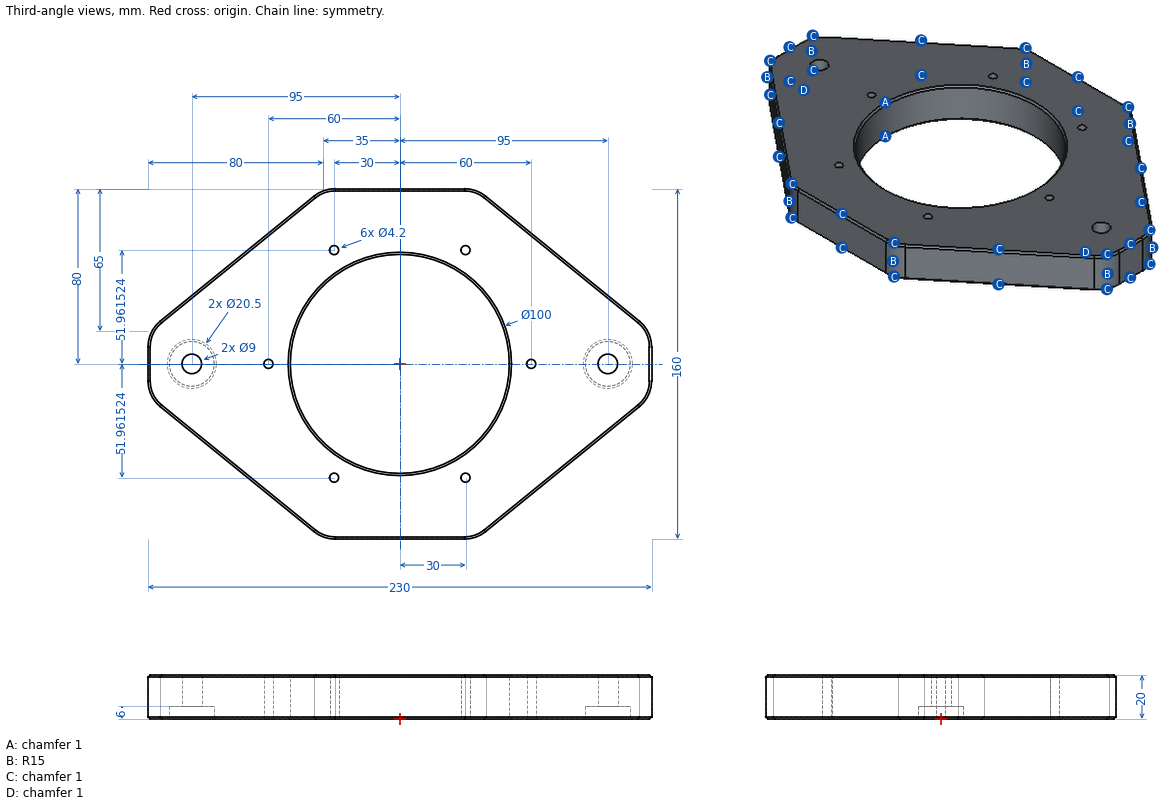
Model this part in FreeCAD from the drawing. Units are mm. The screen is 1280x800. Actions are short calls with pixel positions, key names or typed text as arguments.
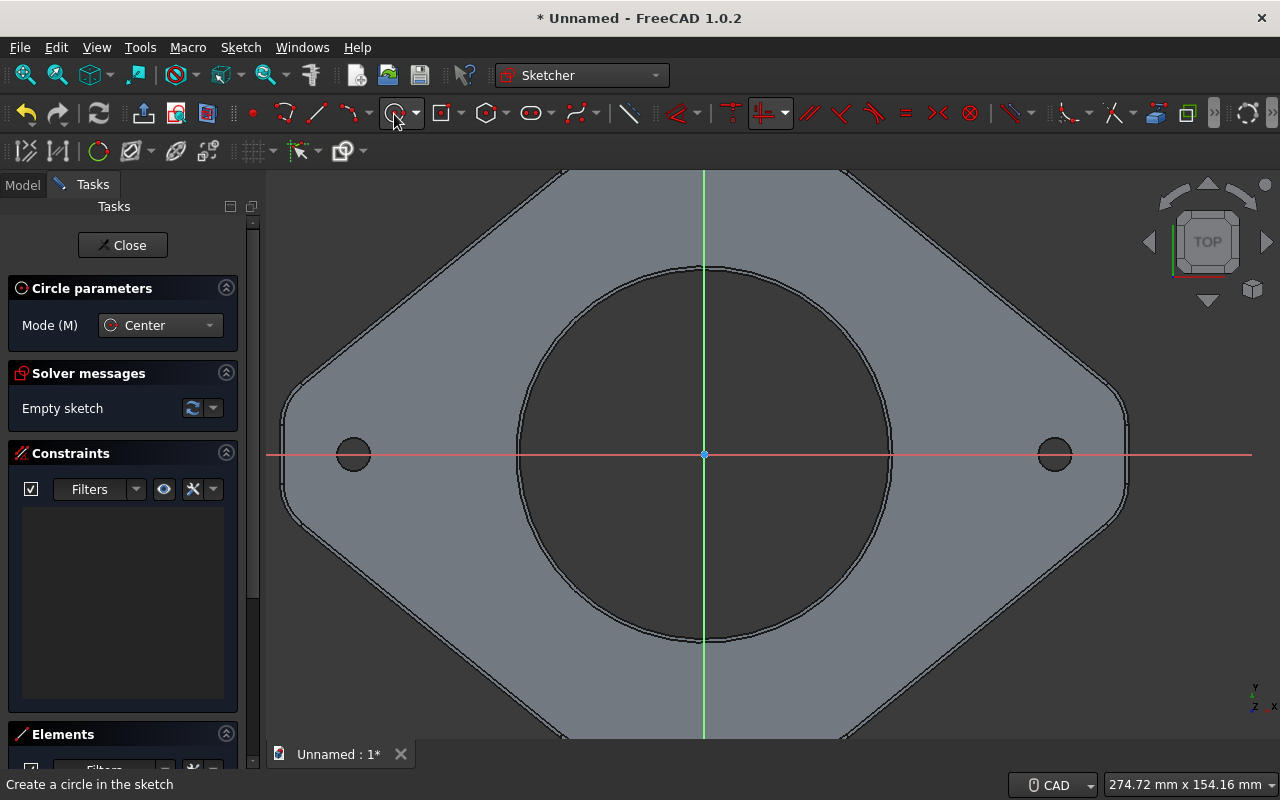
scroll(594, 263, up, 6)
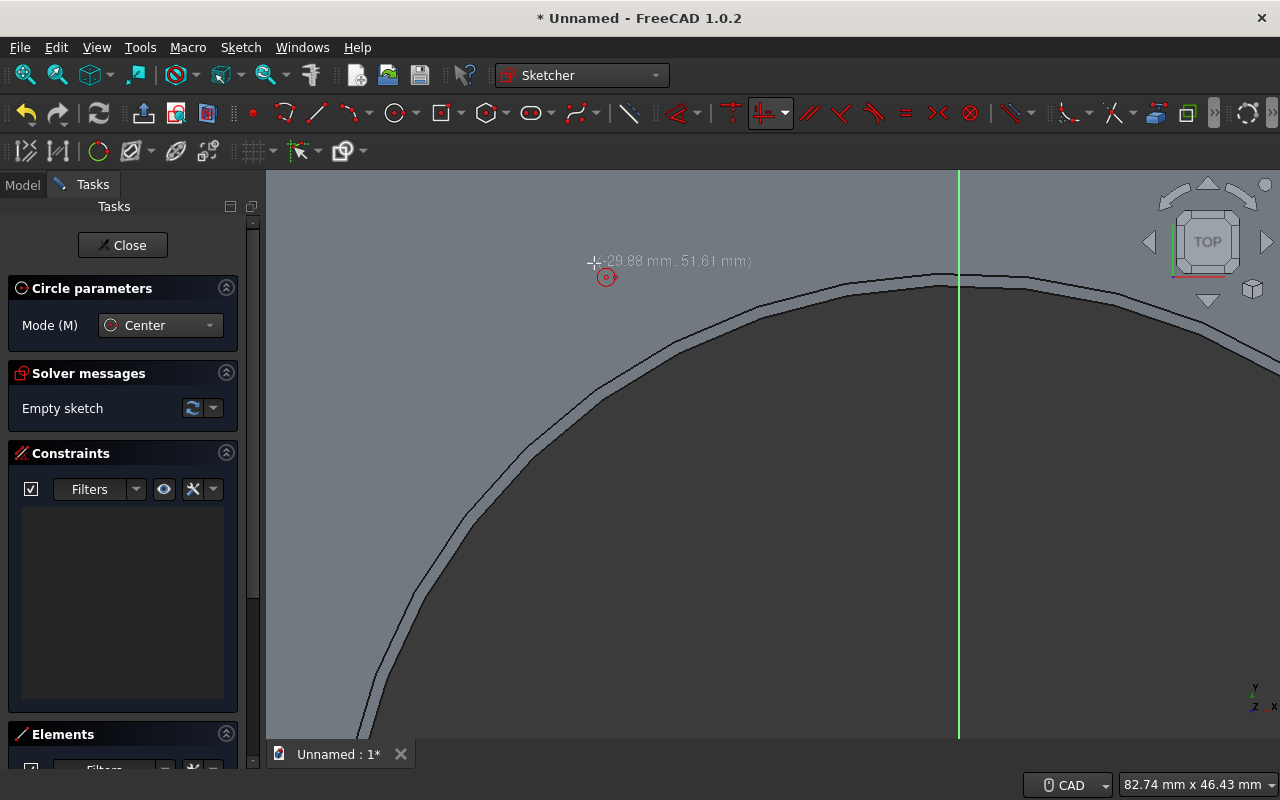
click(592, 262)
move(610, 243)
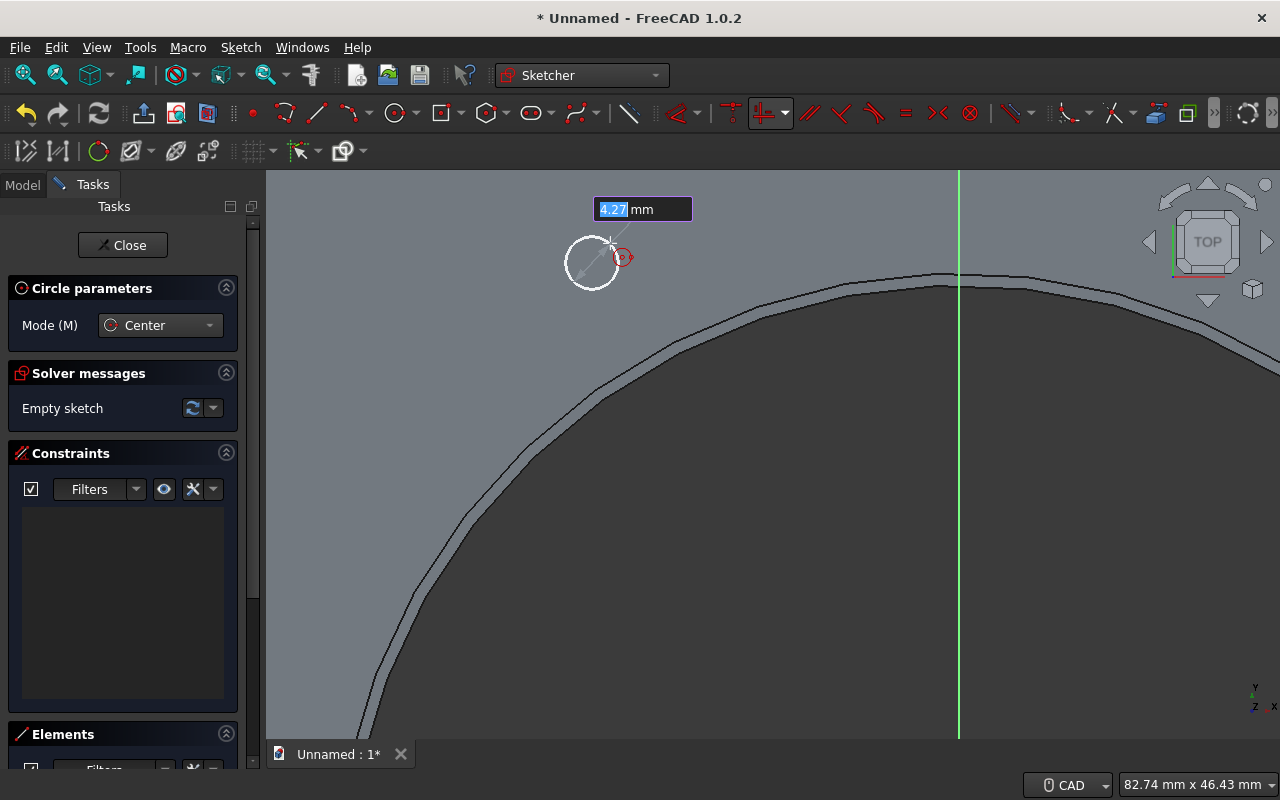
text(4.2)
key(Return)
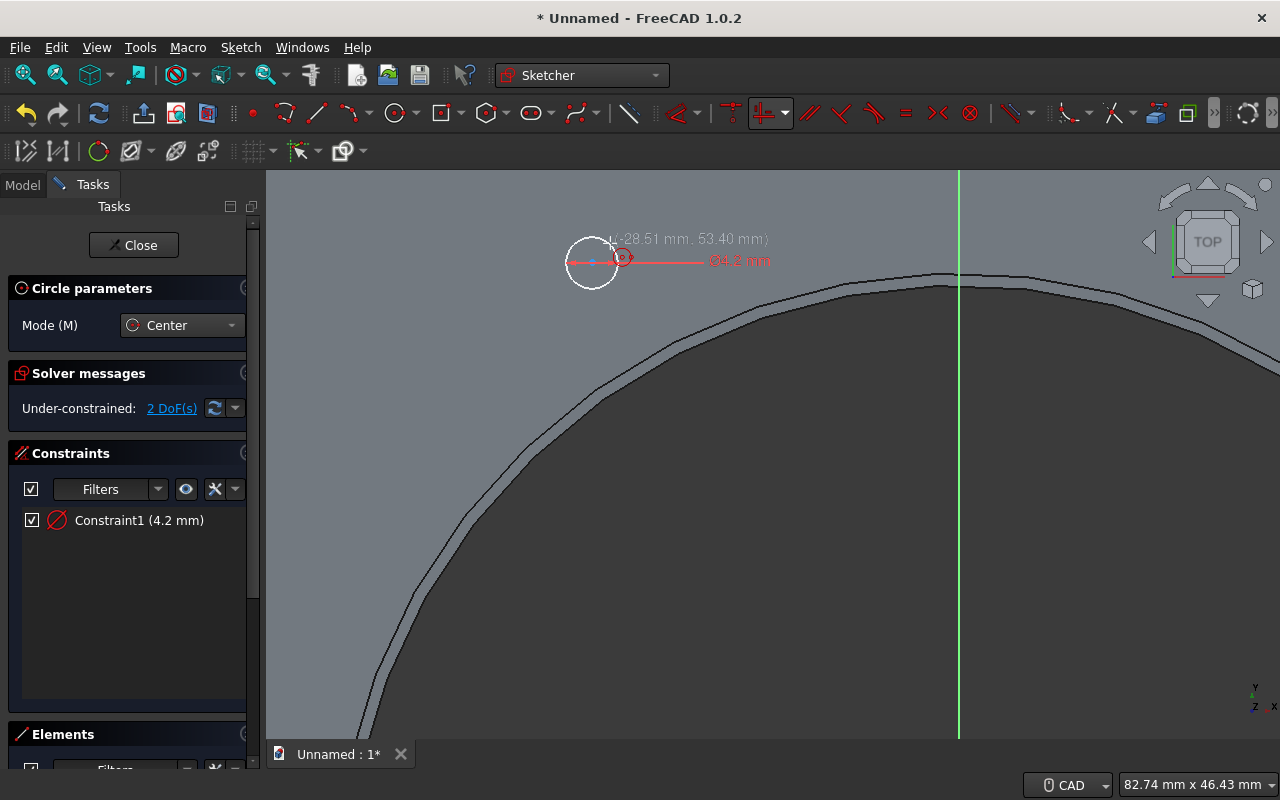
scroll(595, 263, down, 6)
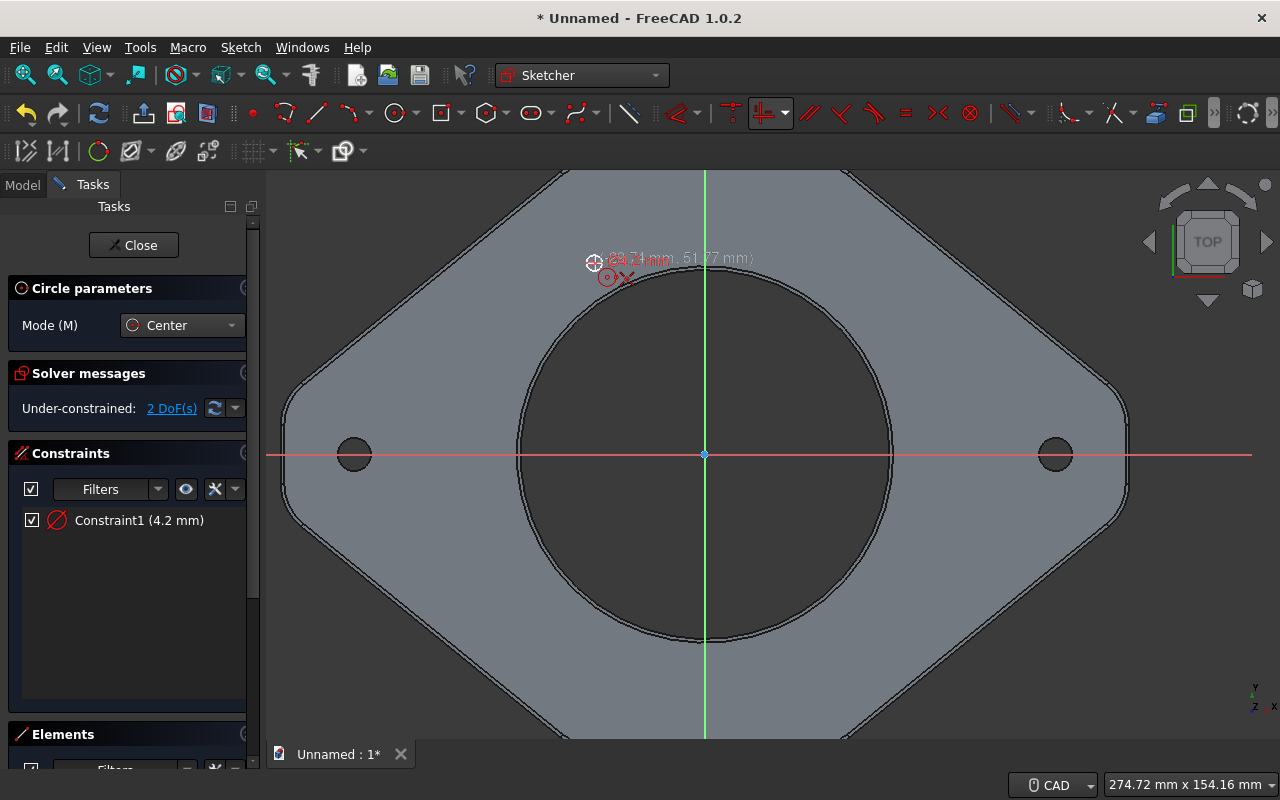
scroll(484, 454, up, 6)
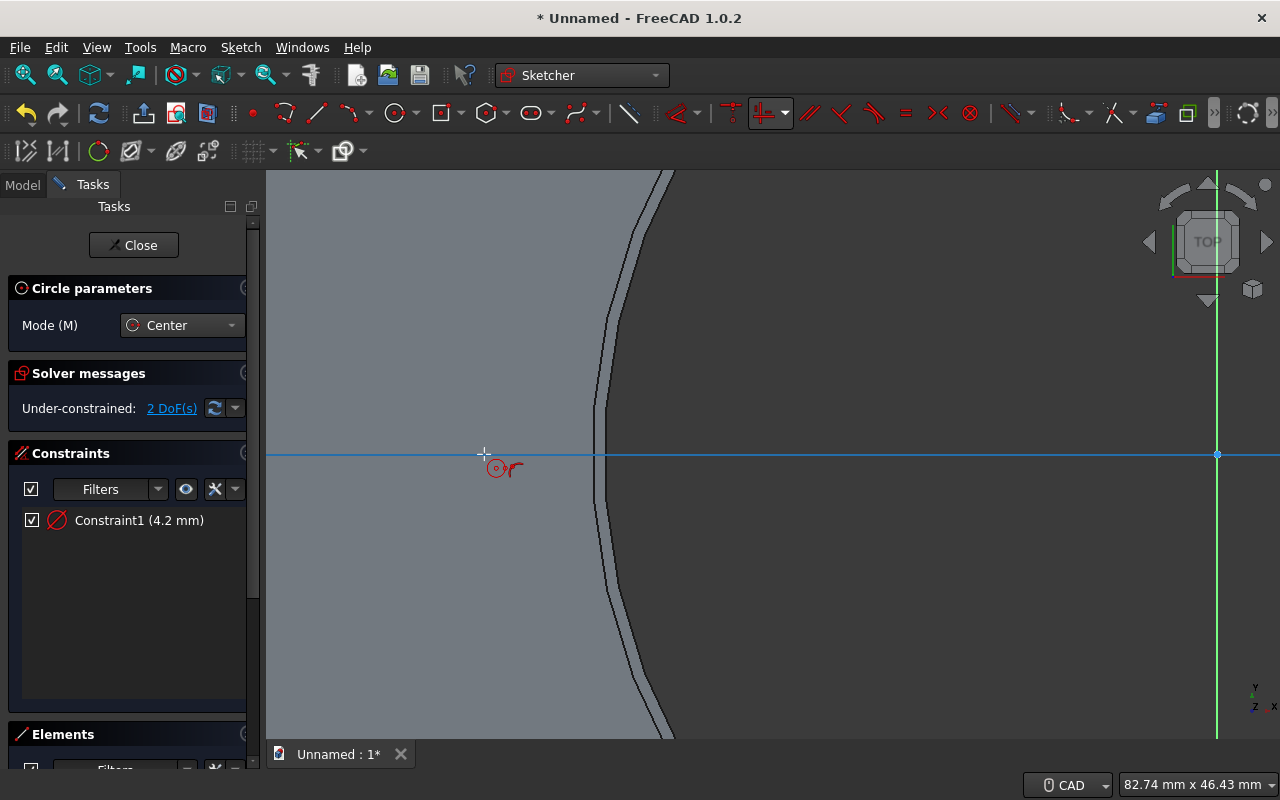
click(482, 454)
move(500, 436)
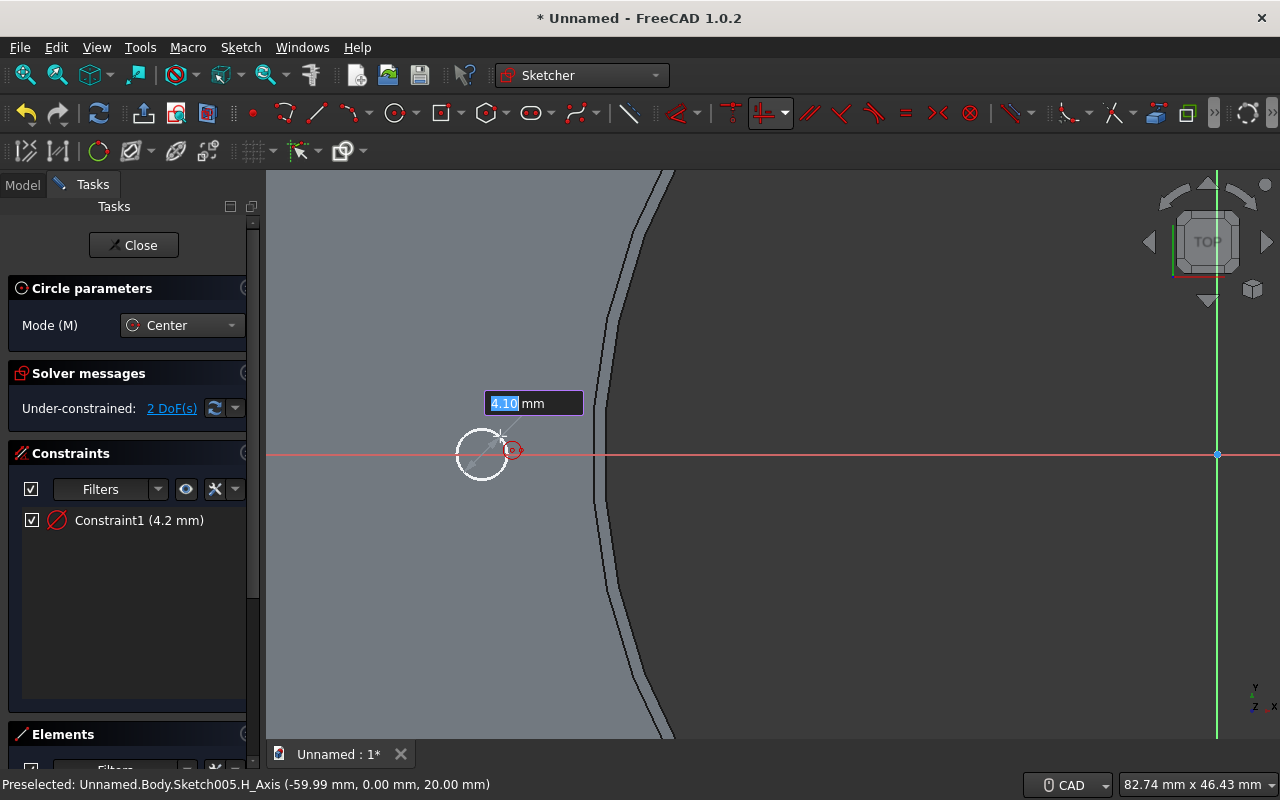
text(4.2)
key(Return)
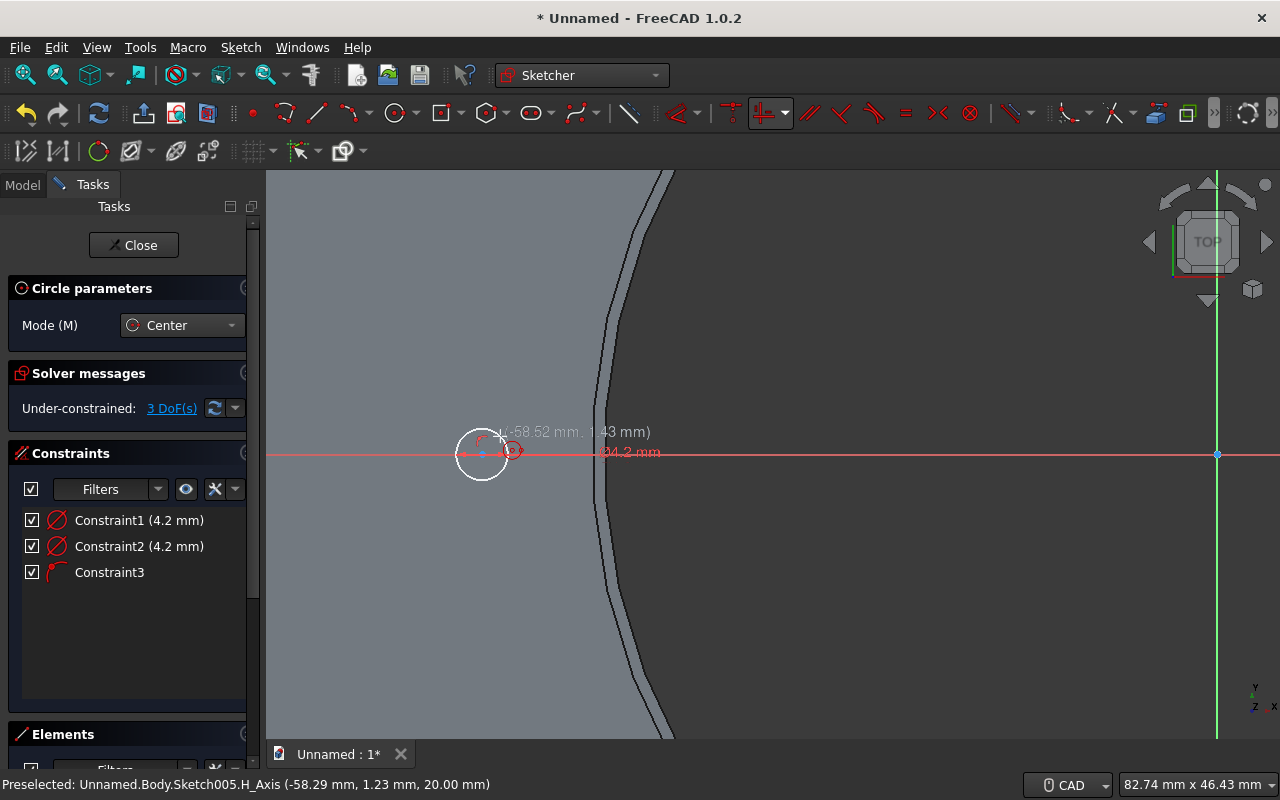
scroll(484, 455, down, 6)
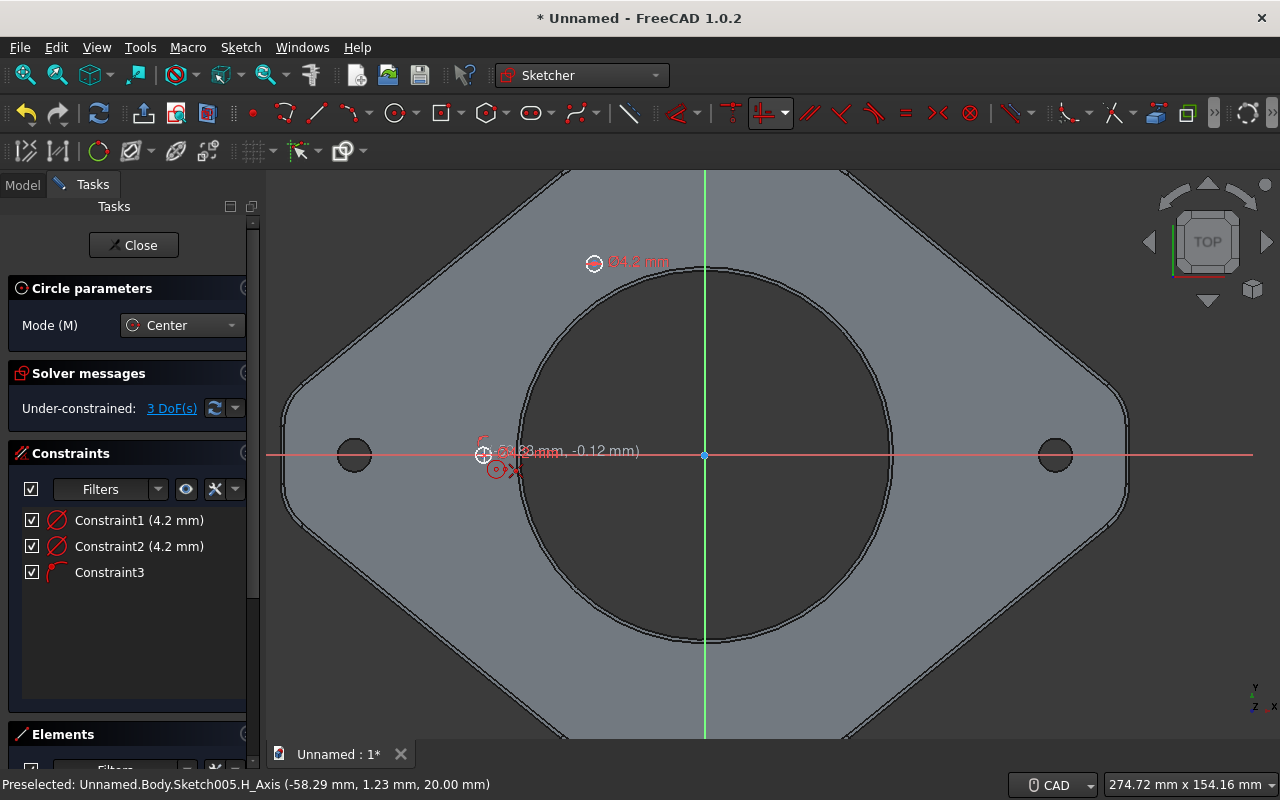
scroll(594, 647, up, 6)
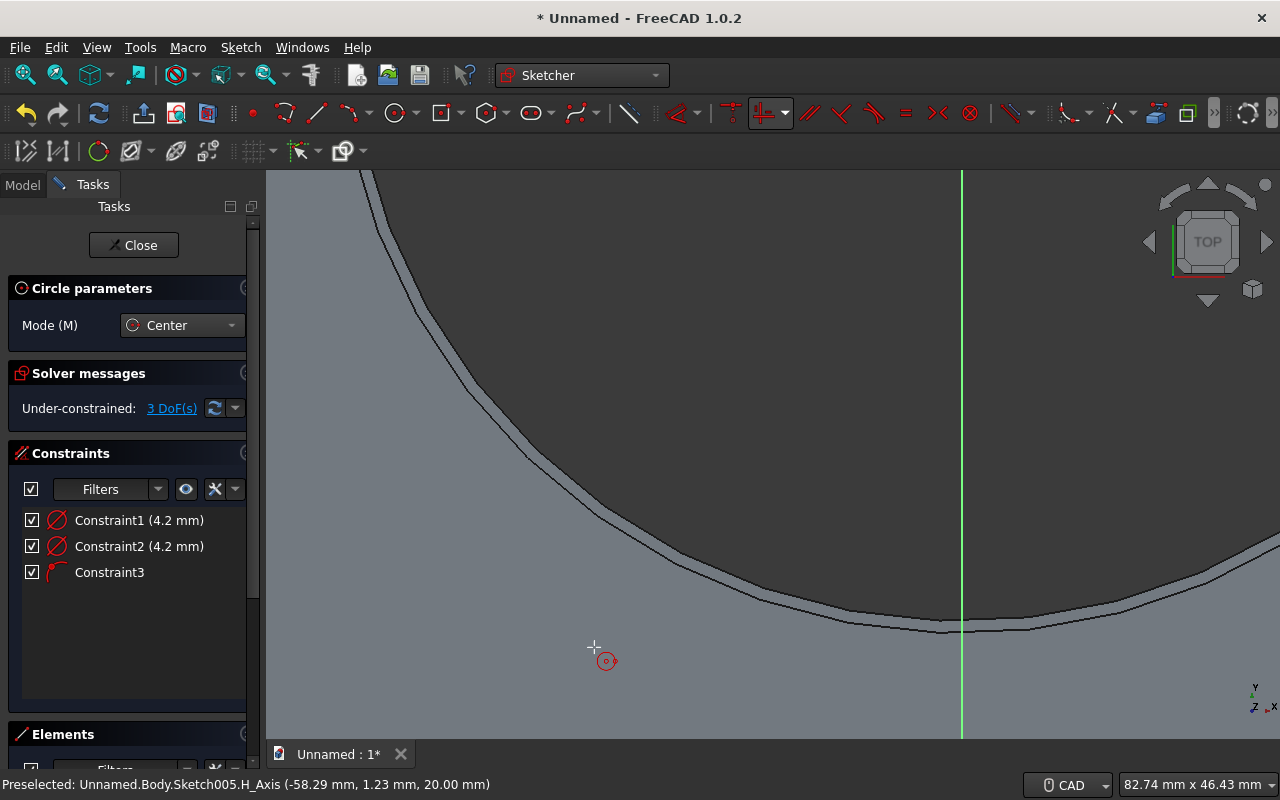
click(594, 645)
move(612, 627)